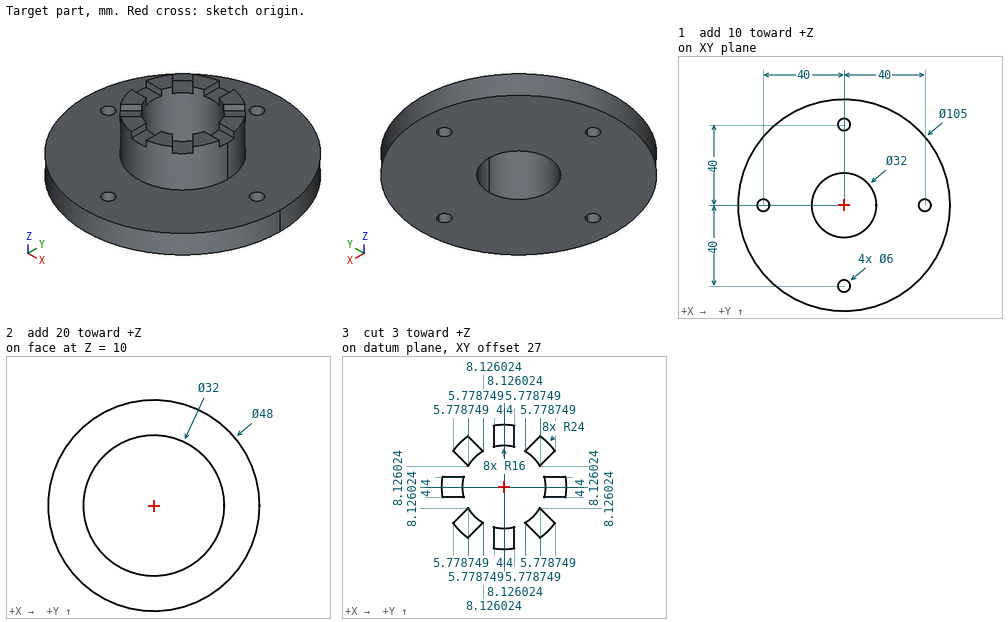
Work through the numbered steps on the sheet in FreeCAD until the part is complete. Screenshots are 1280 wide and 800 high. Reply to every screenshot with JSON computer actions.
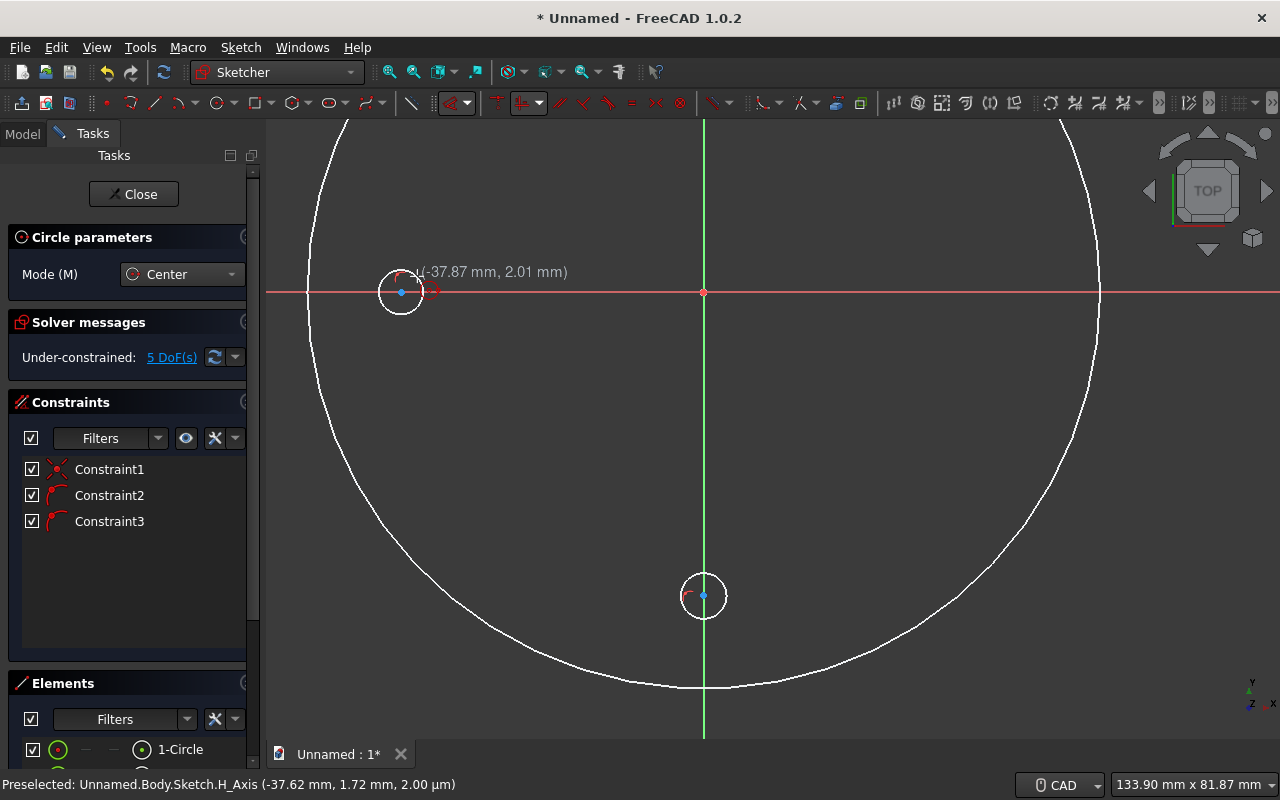
{"action": "left_click", "coordinate": [704, 292]}
{"action": "left_click", "coordinate": [789, 207]}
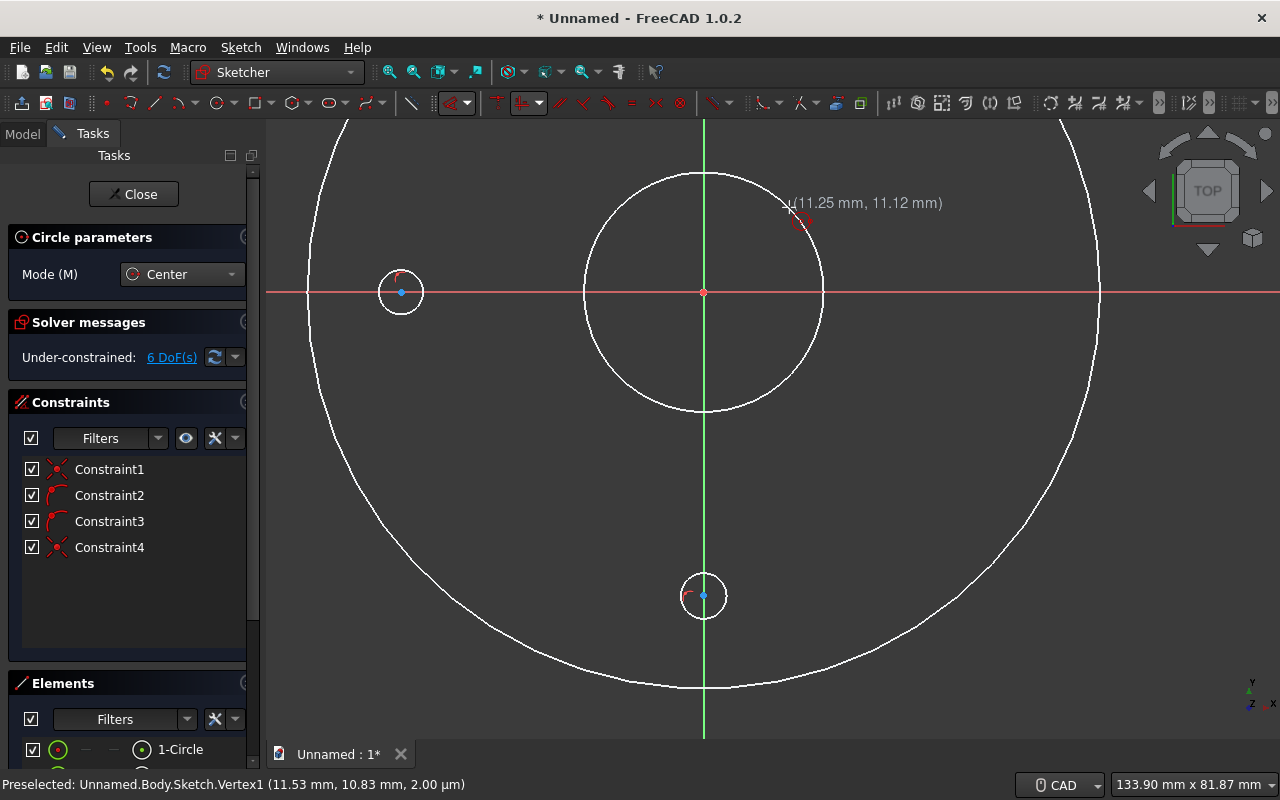
{"action": "left_click", "coordinate": [1007, 292]}
{"action": "left_click", "coordinate": [1023, 276]}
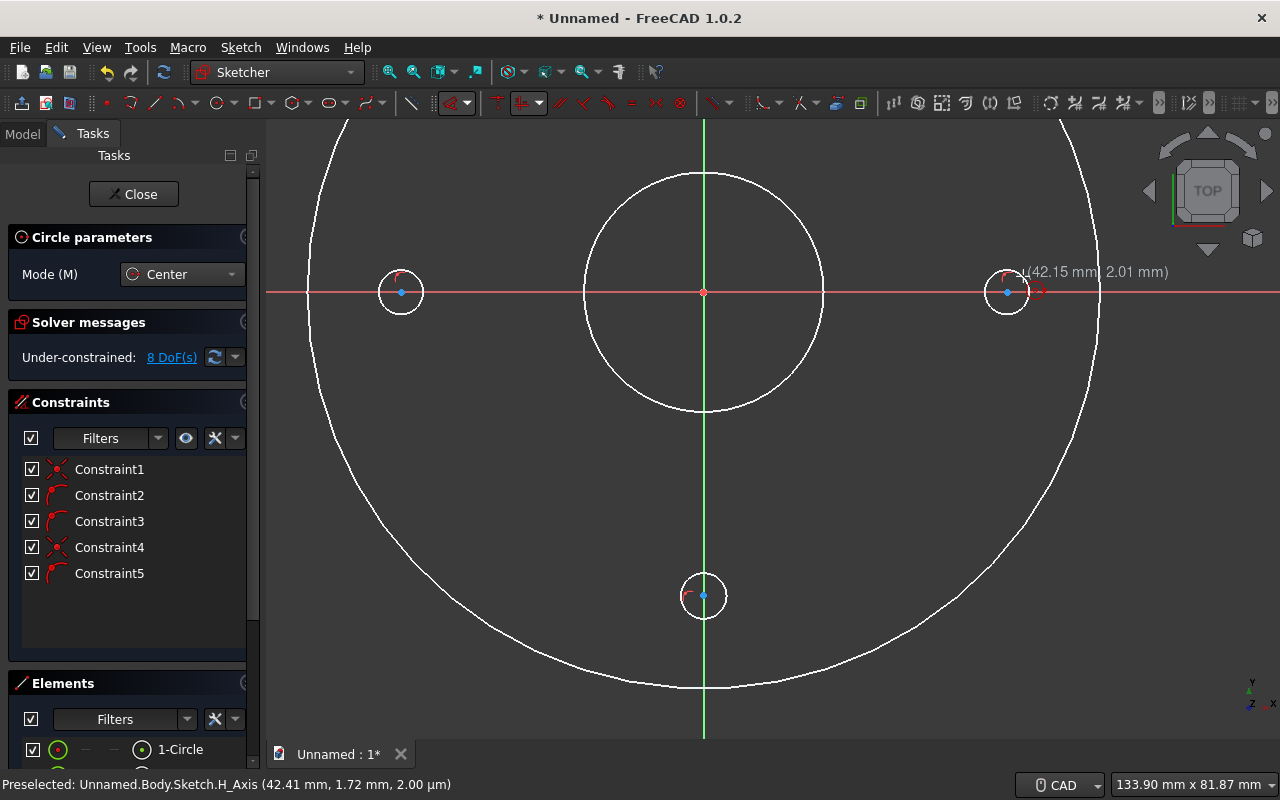
{"action": "scroll", "coordinate": [705, 595], "scroll_direction": "down", "scroll_amount": 3}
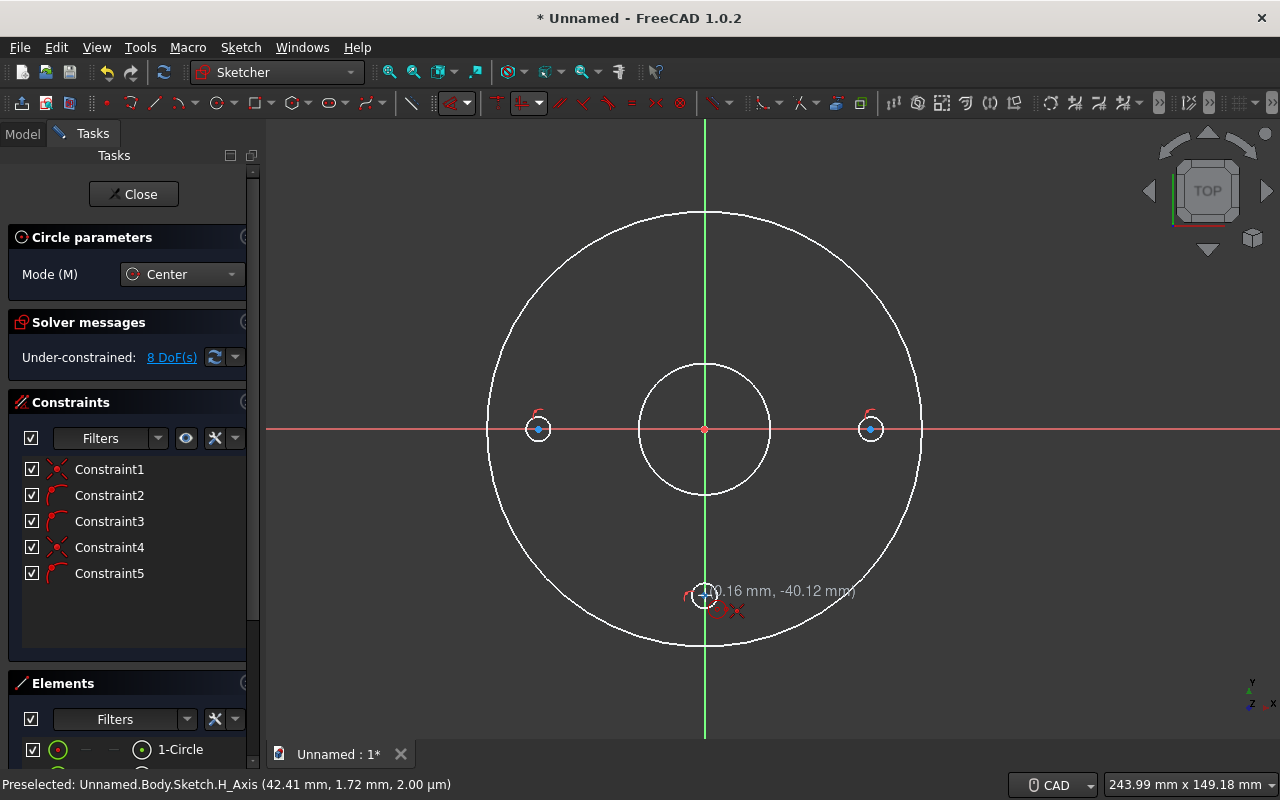
{"action": "scroll", "coordinate": [705, 263], "scroll_direction": "up", "scroll_amount": 3}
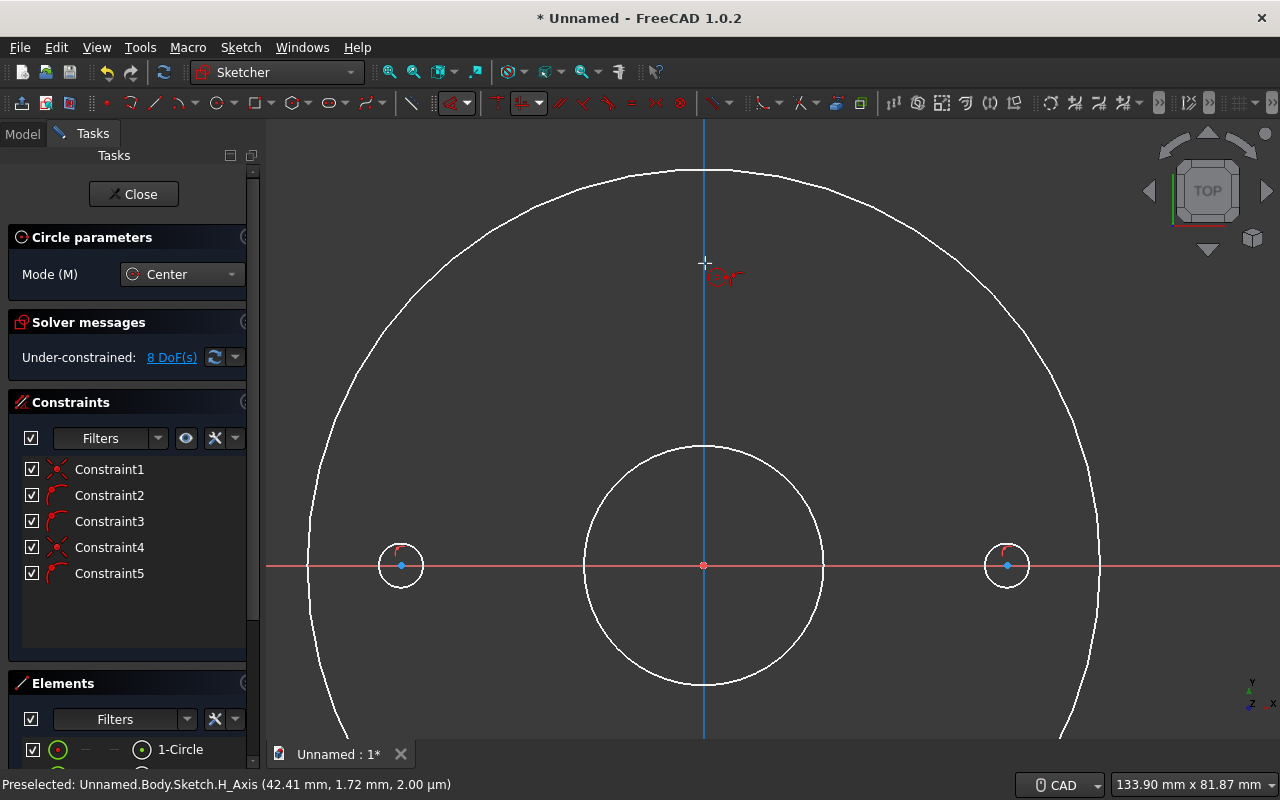
{"action": "left_click", "coordinate": [704, 263]}
{"action": "left_click", "coordinate": [720, 247]}
{"action": "key", "text": "Escape"}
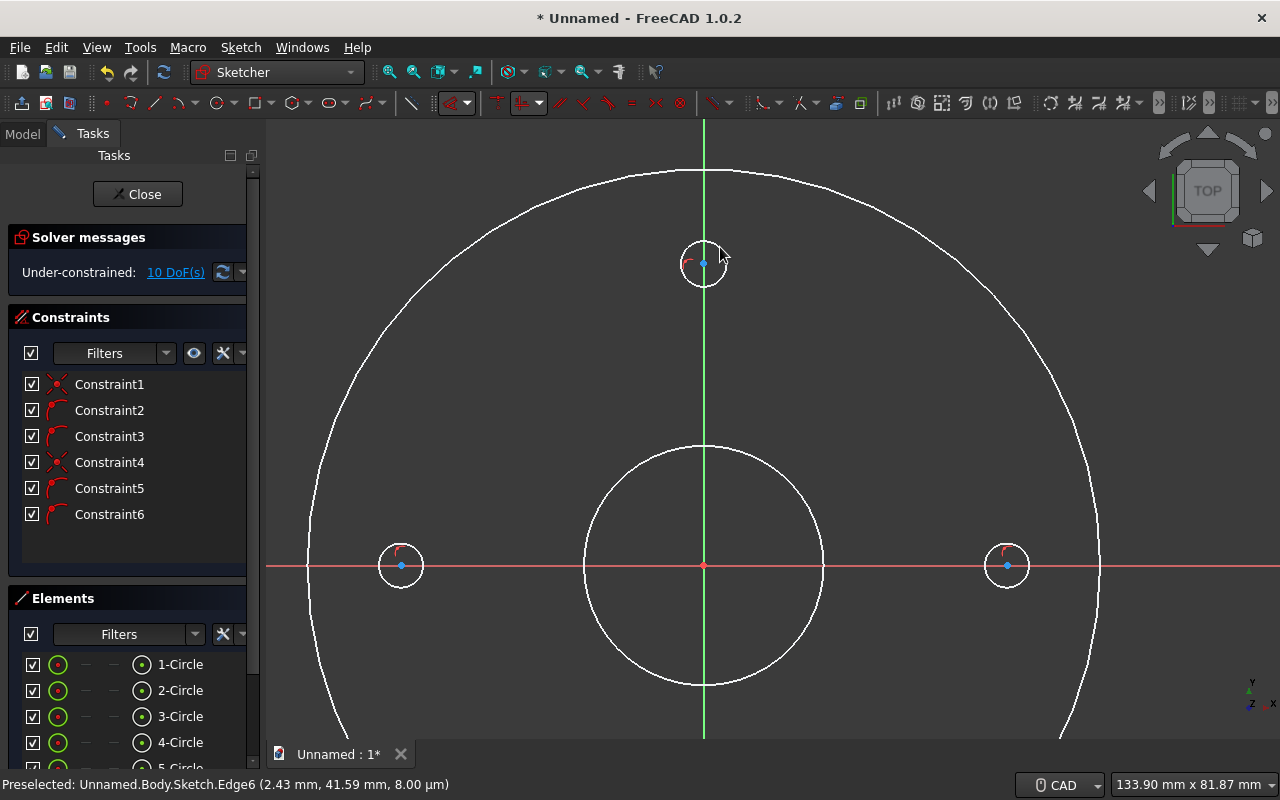
{"action": "scroll", "coordinate": [705, 263], "scroll_direction": "down", "scroll_amount": 3}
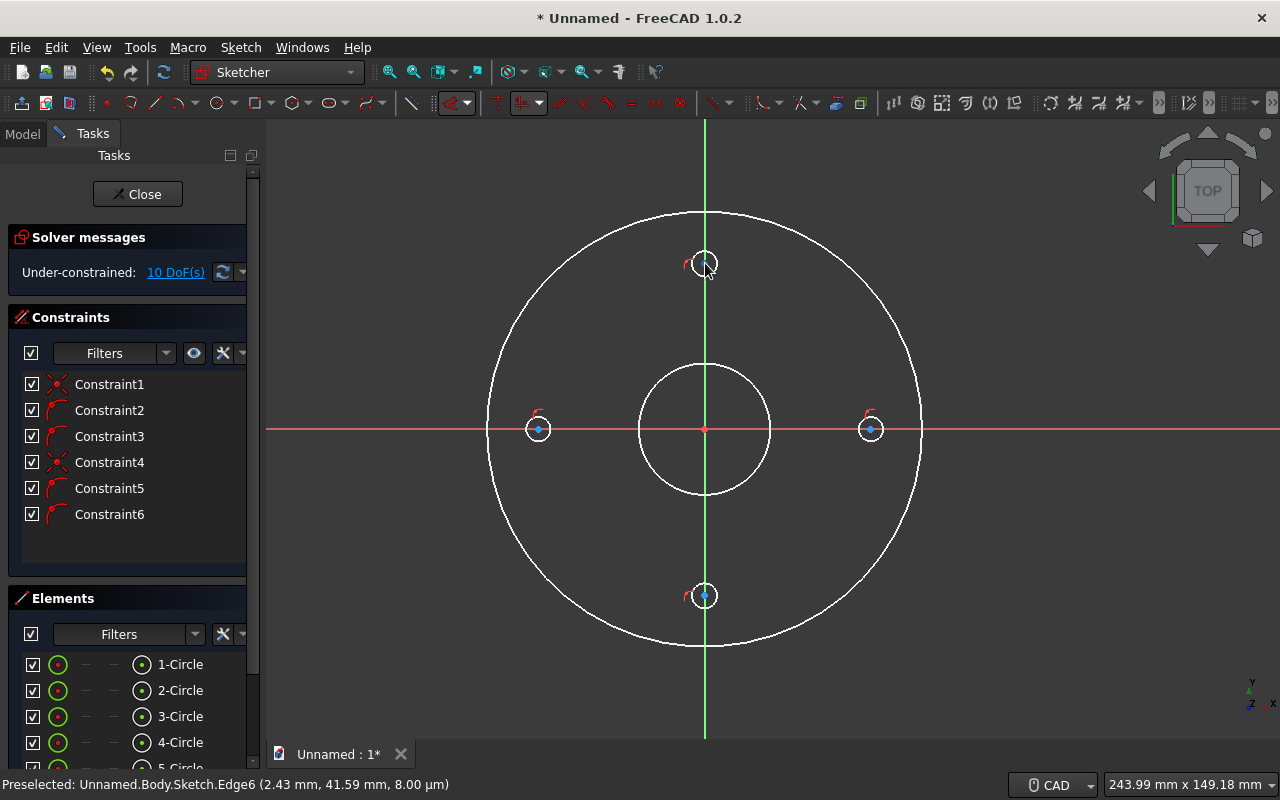
{"action": "scroll", "coordinate": [713, 587], "scroll_direction": "up", "scroll_amount": 3}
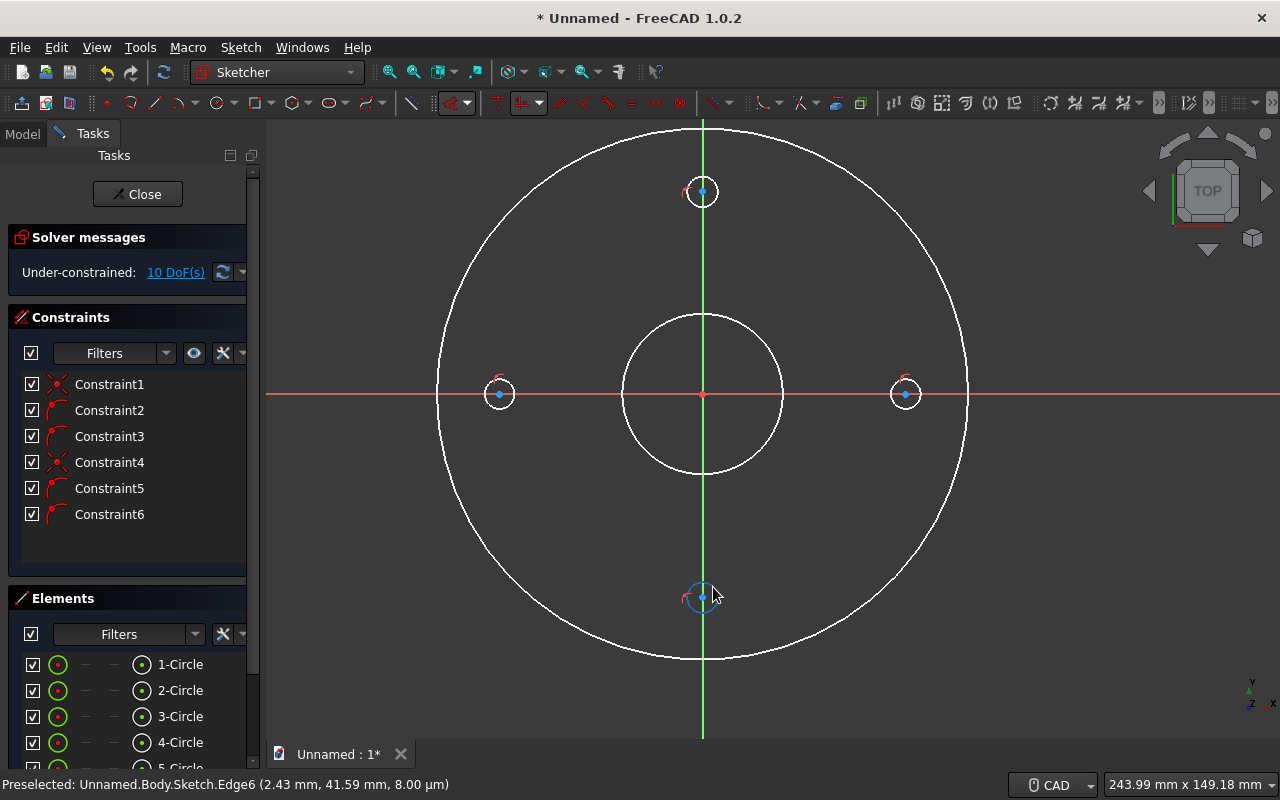
{"action": "left_click", "coordinate": [713, 586]}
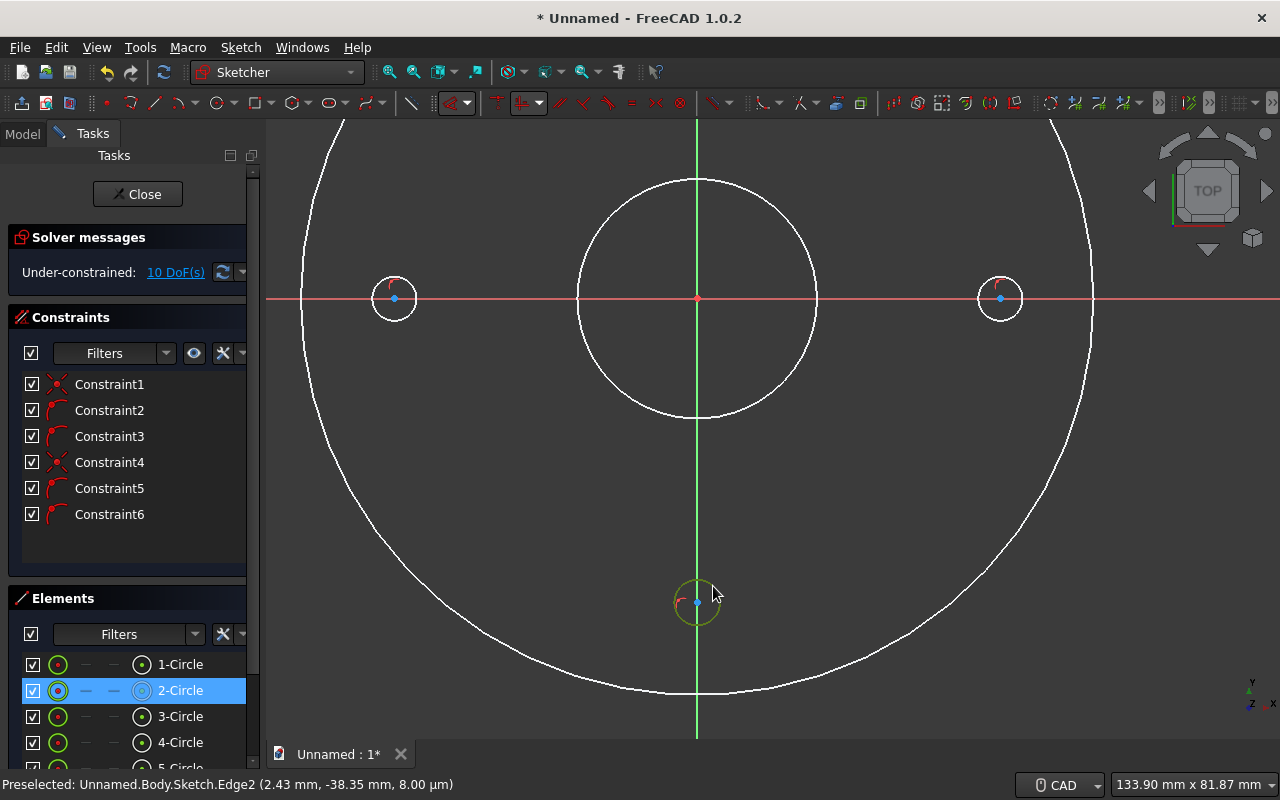
{"action": "left_click", "coordinate": [410, 283]}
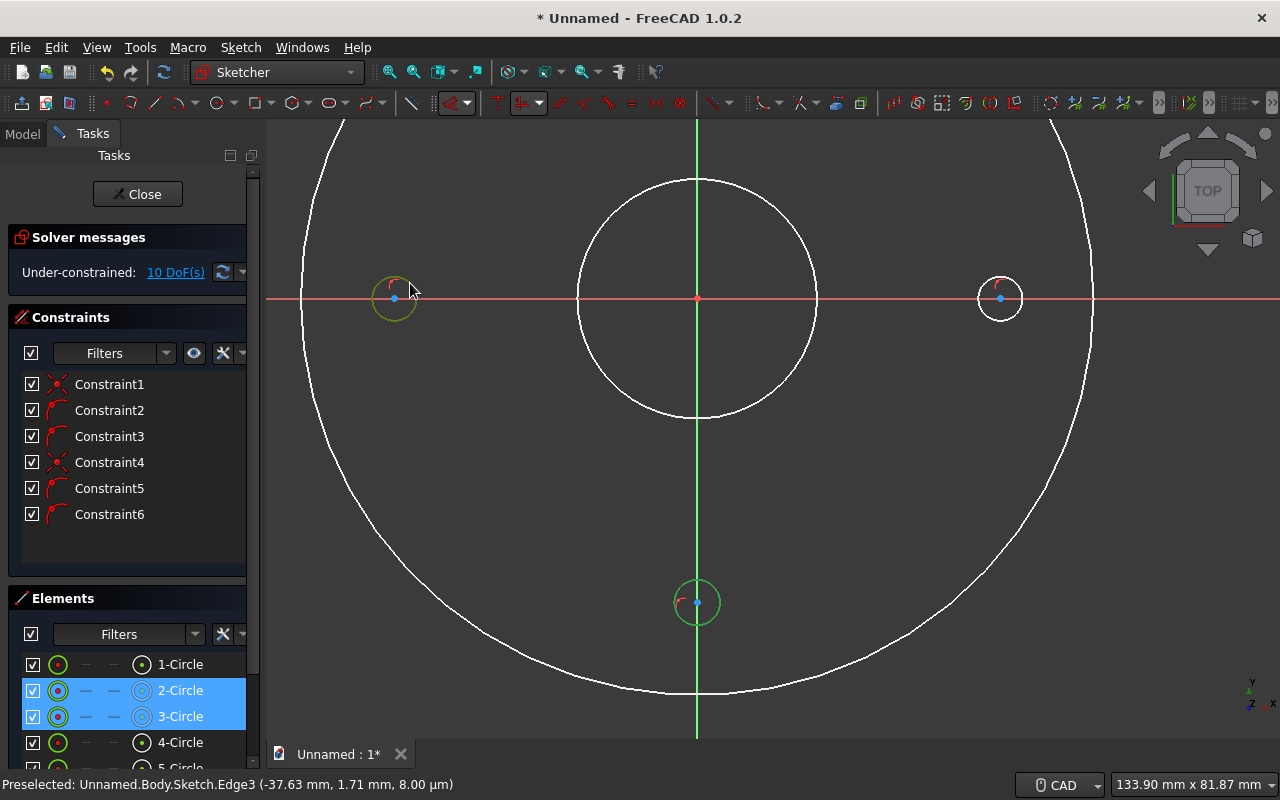
{"action": "left_click", "coordinate": [1016, 283]}